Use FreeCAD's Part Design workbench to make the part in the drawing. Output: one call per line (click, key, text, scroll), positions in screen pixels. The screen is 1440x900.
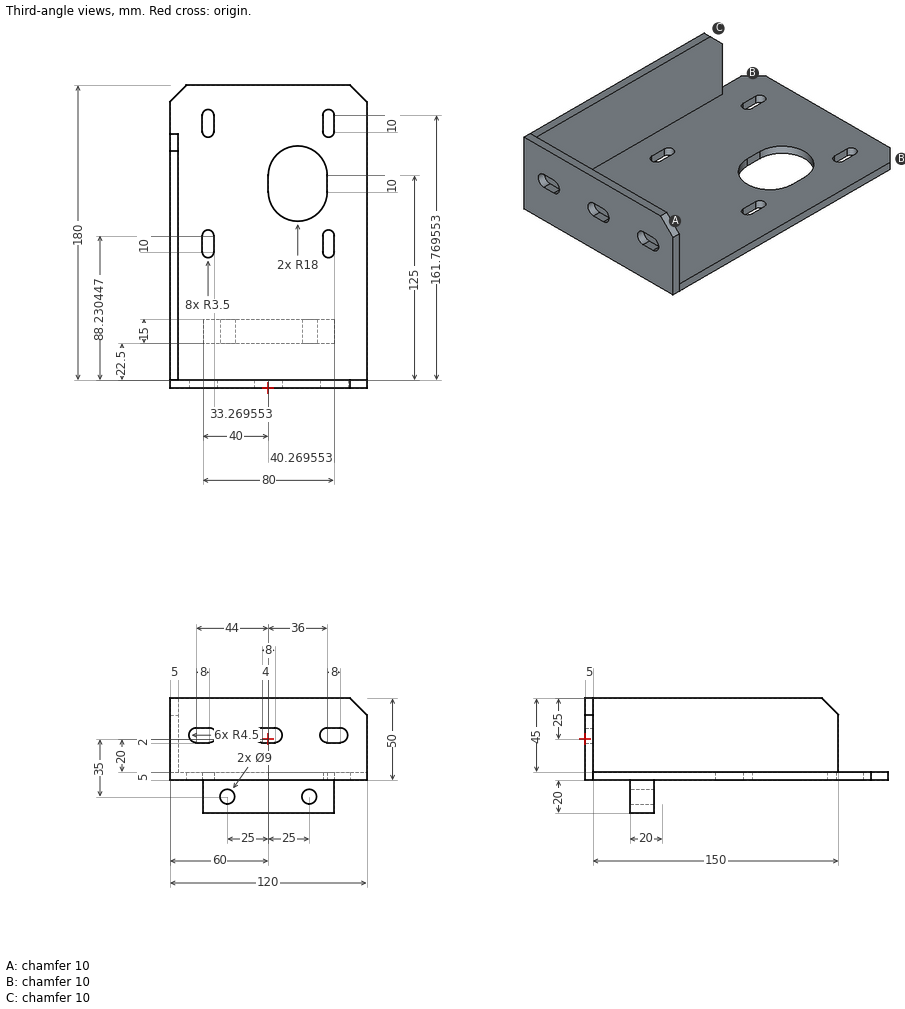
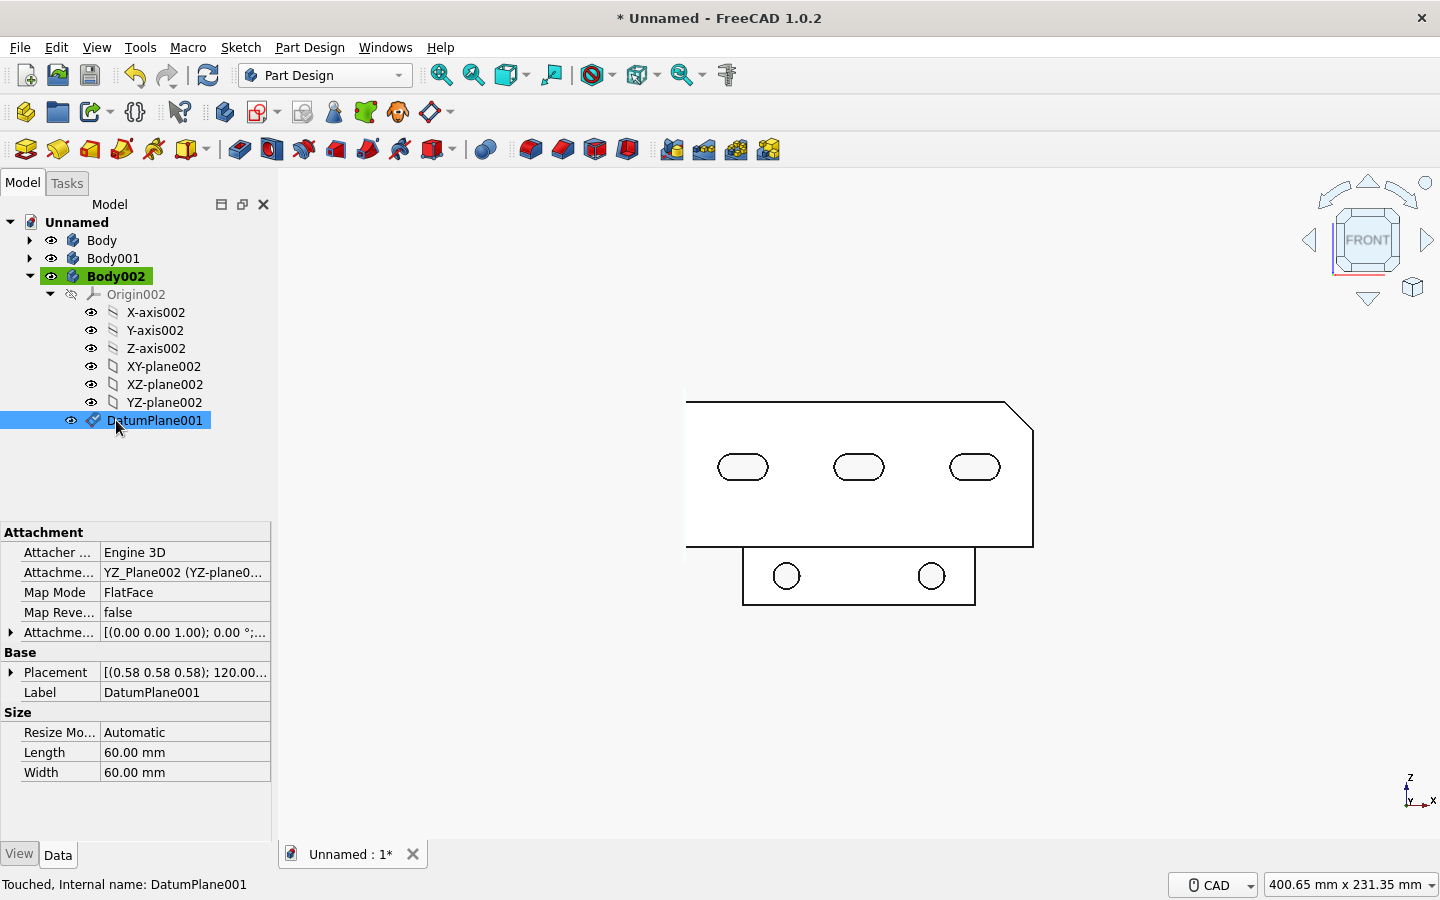
click(258, 112)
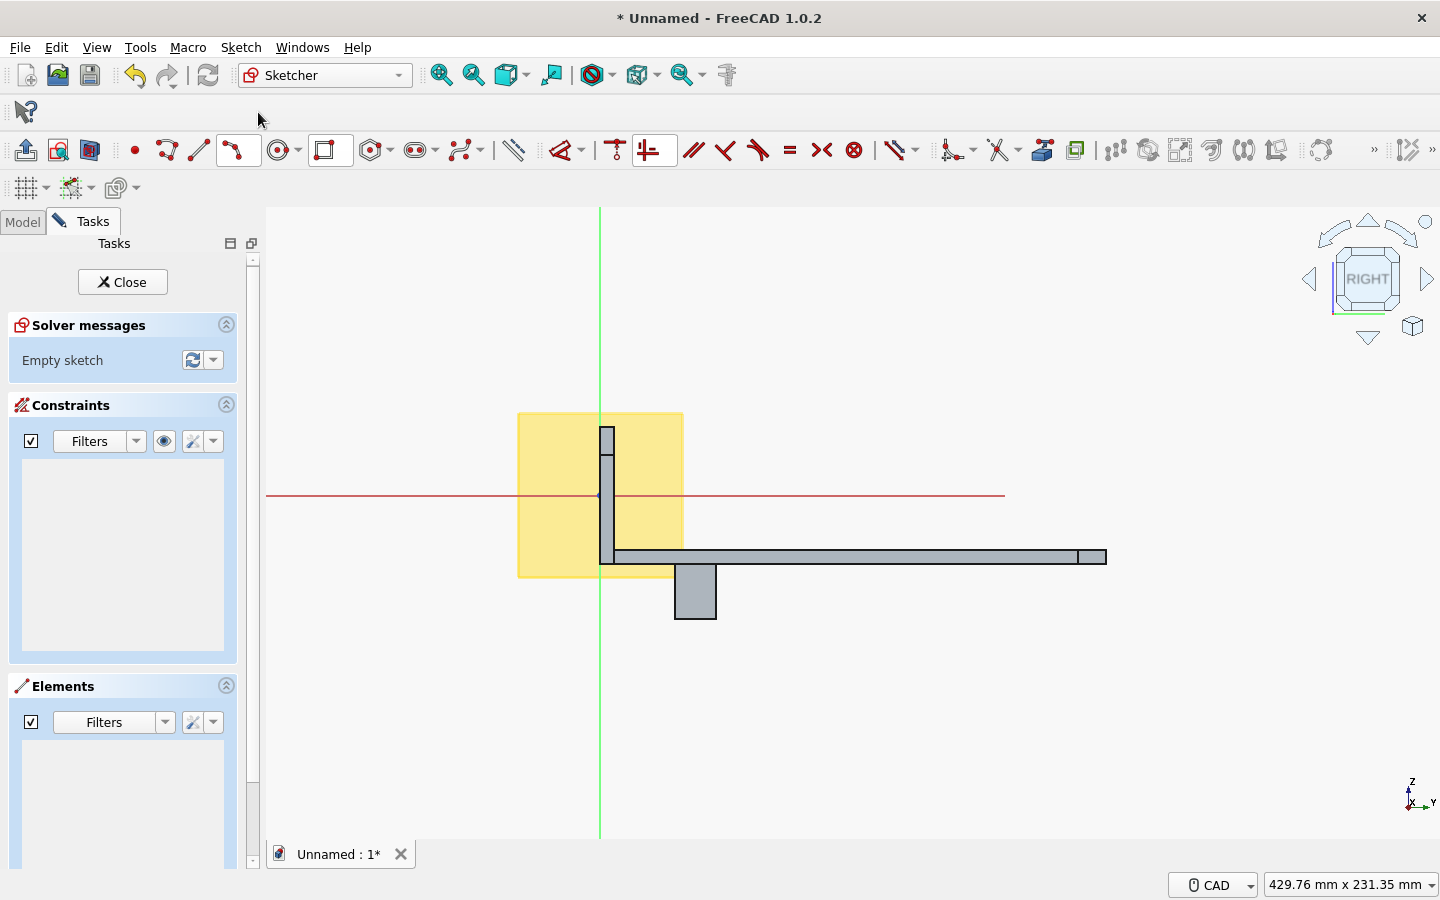
scroll(868, 419, up, 2)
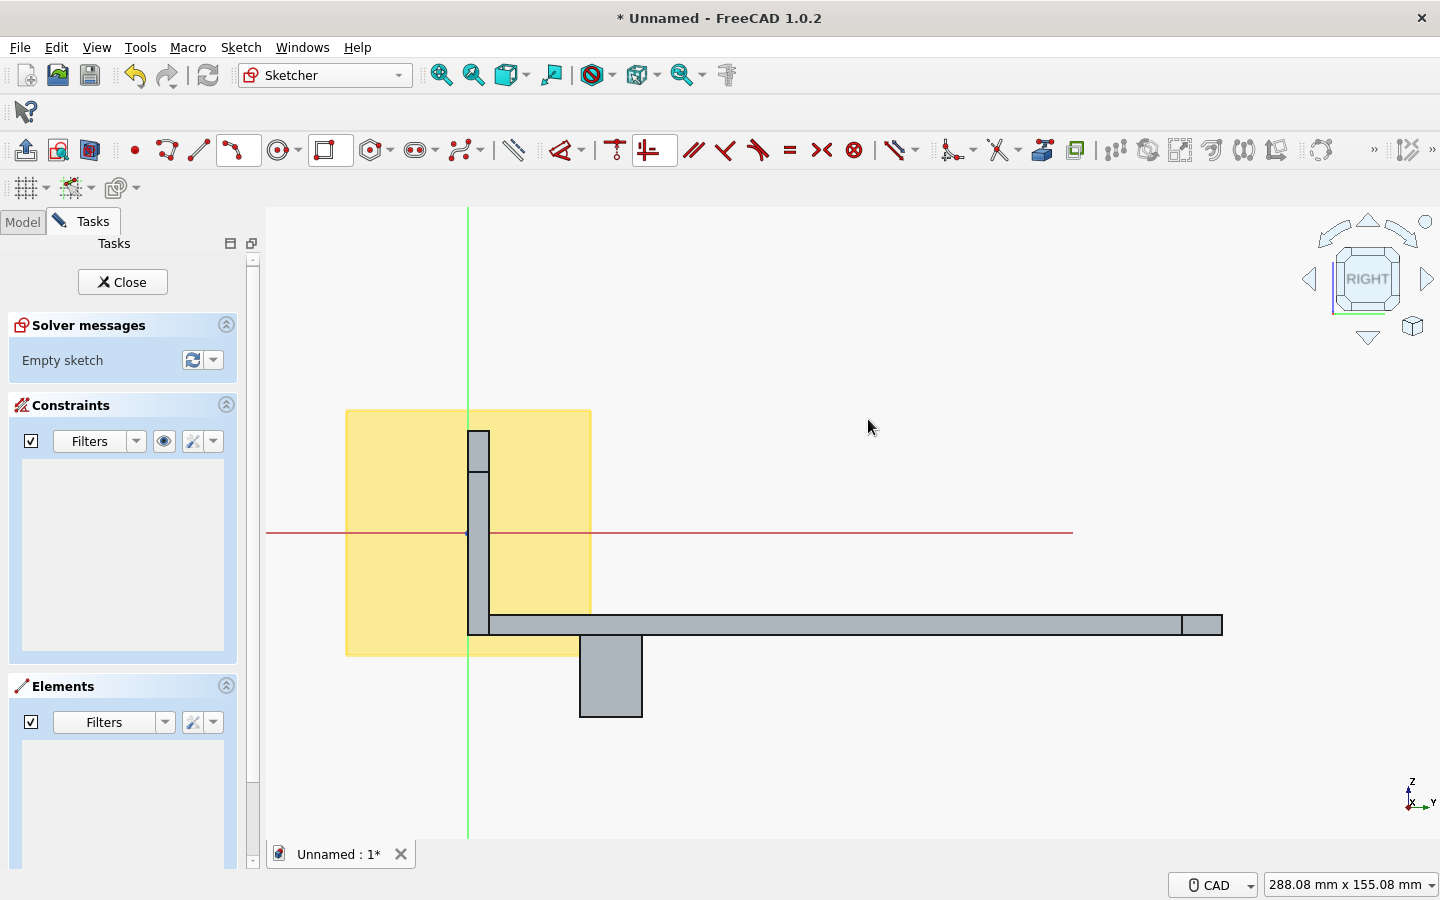
key(g)
key(r)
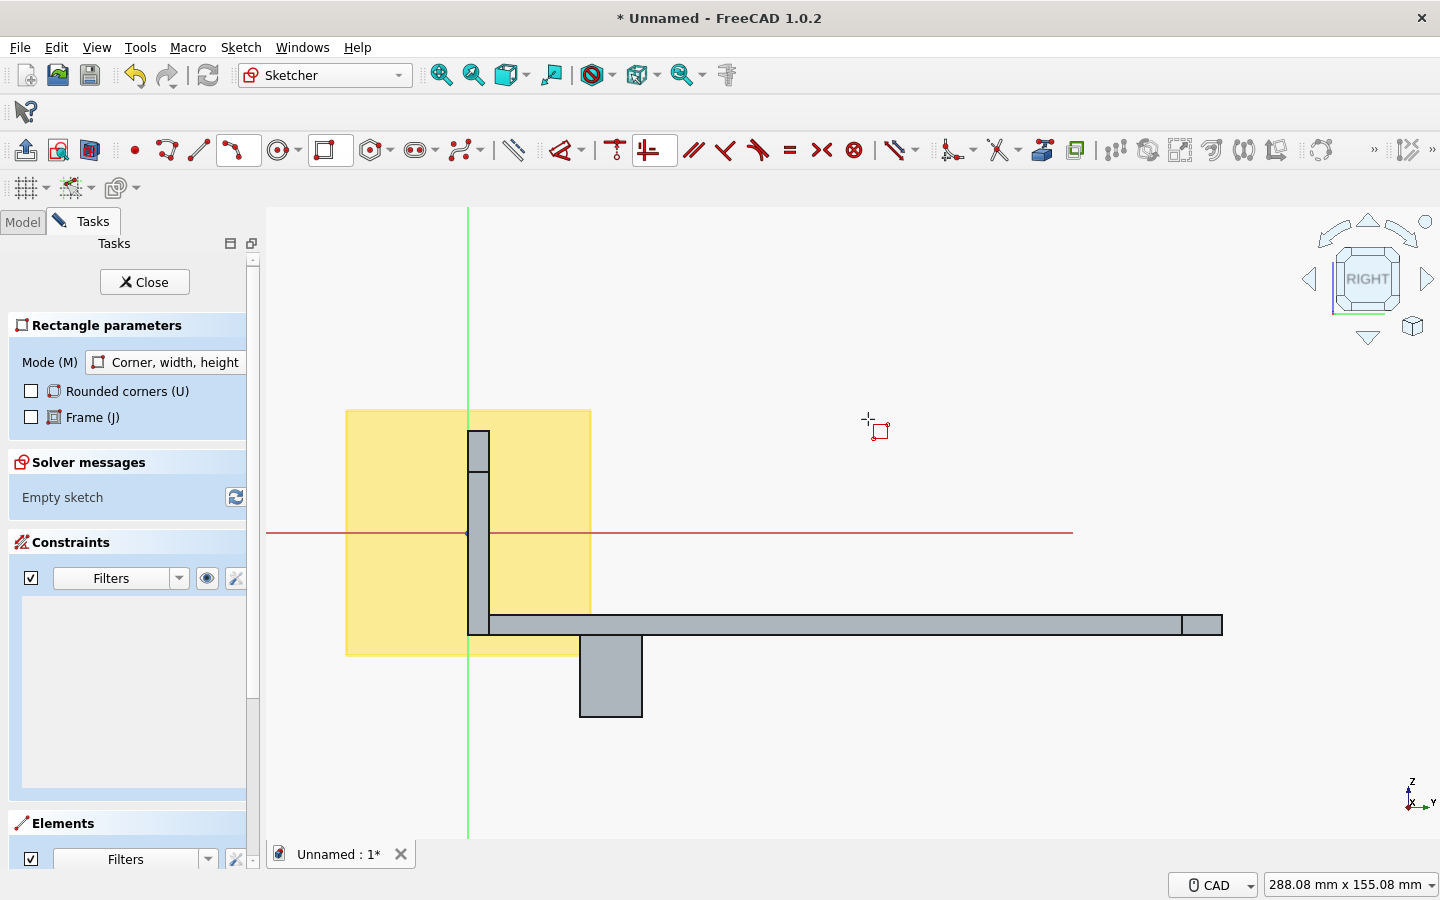
click(489, 431)
click(1100, 615)
key(Escape)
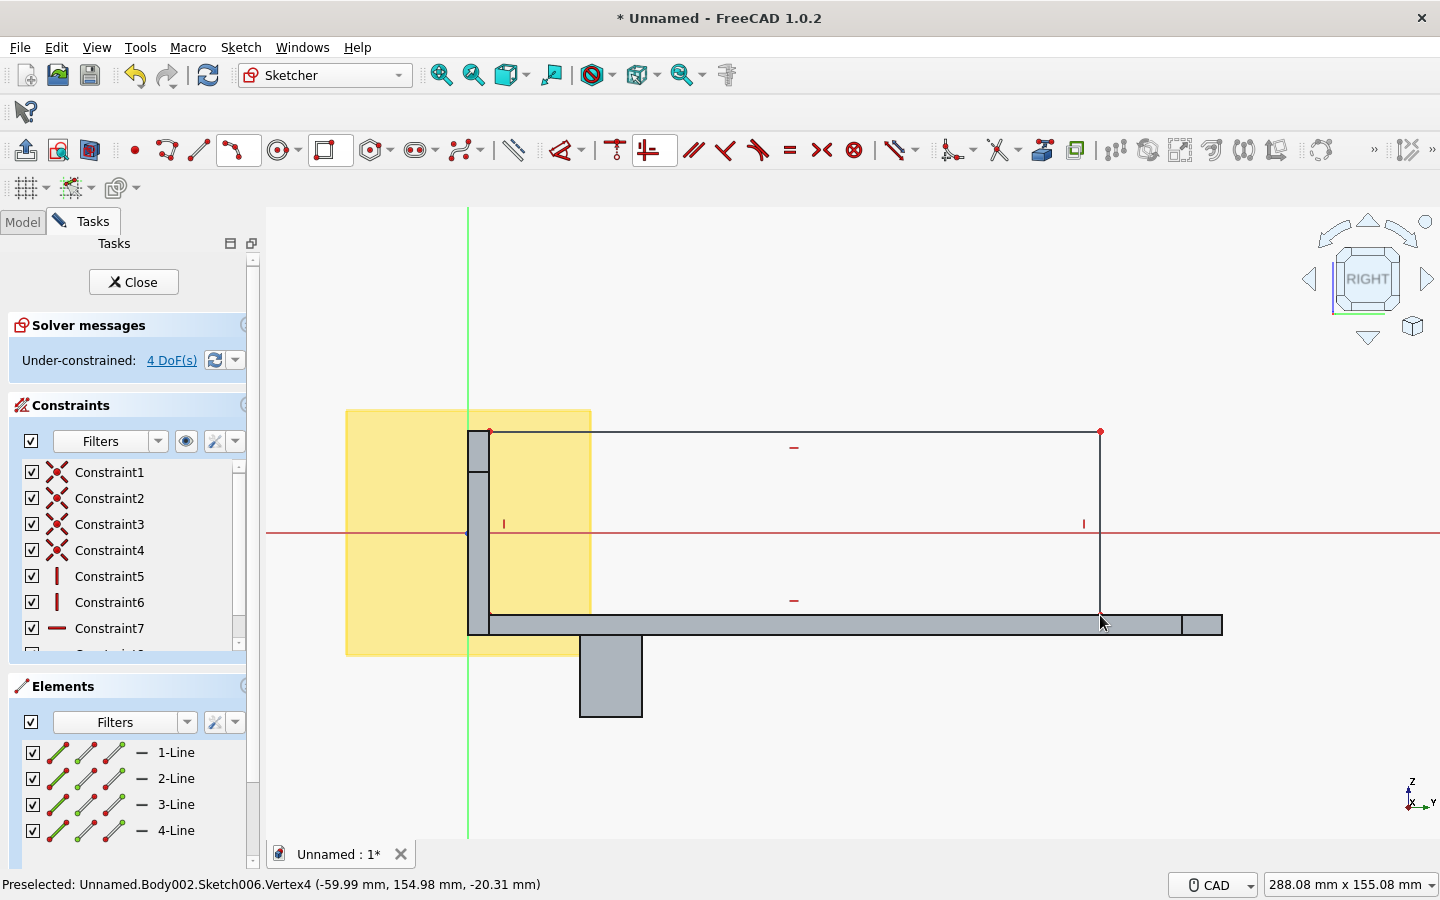
key(d)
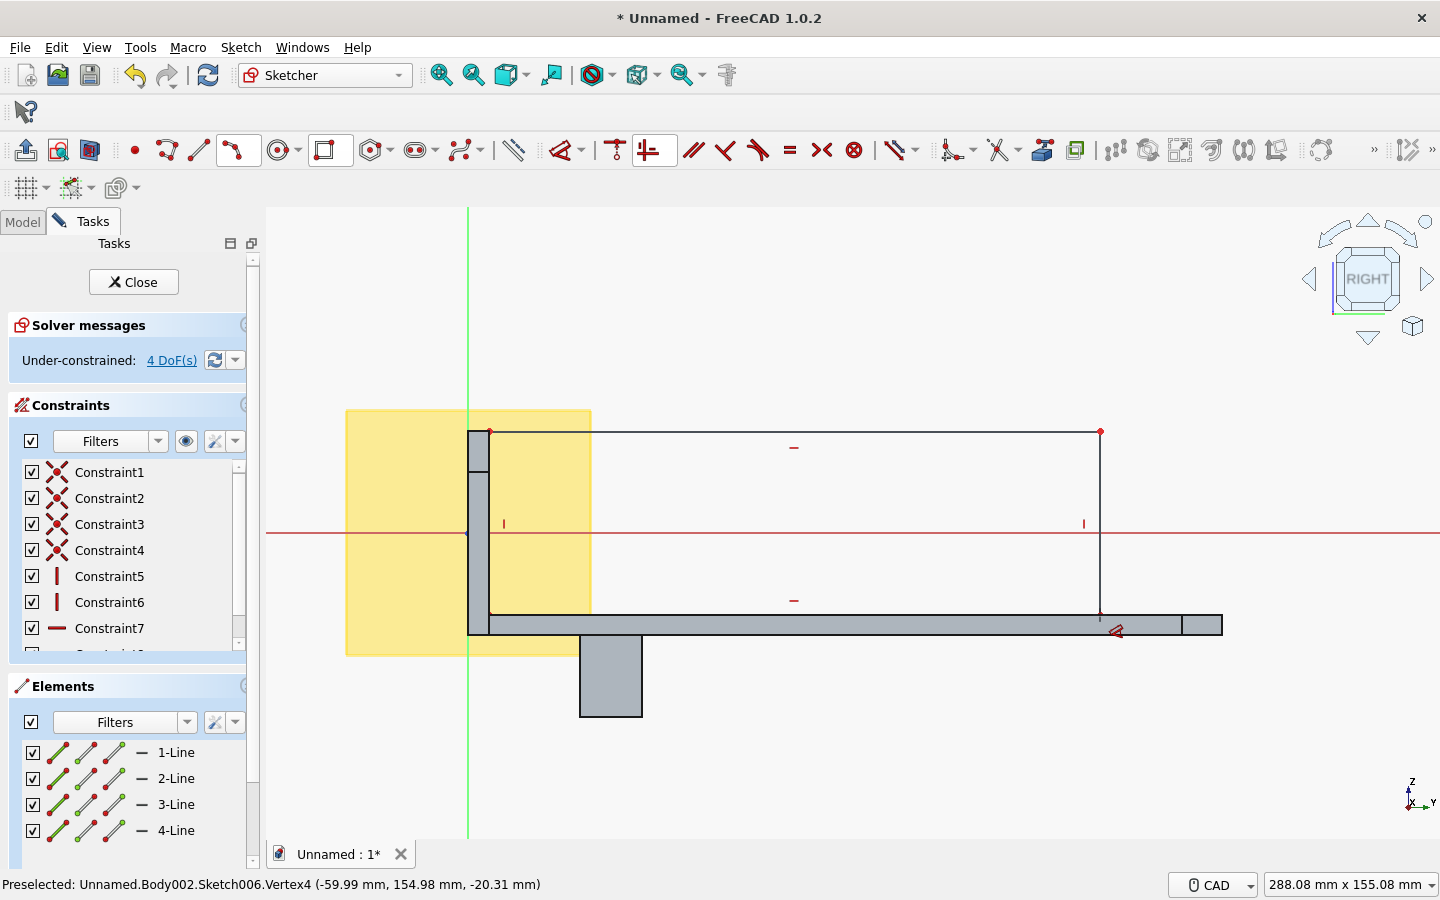
click(489, 487)
click(455, 482)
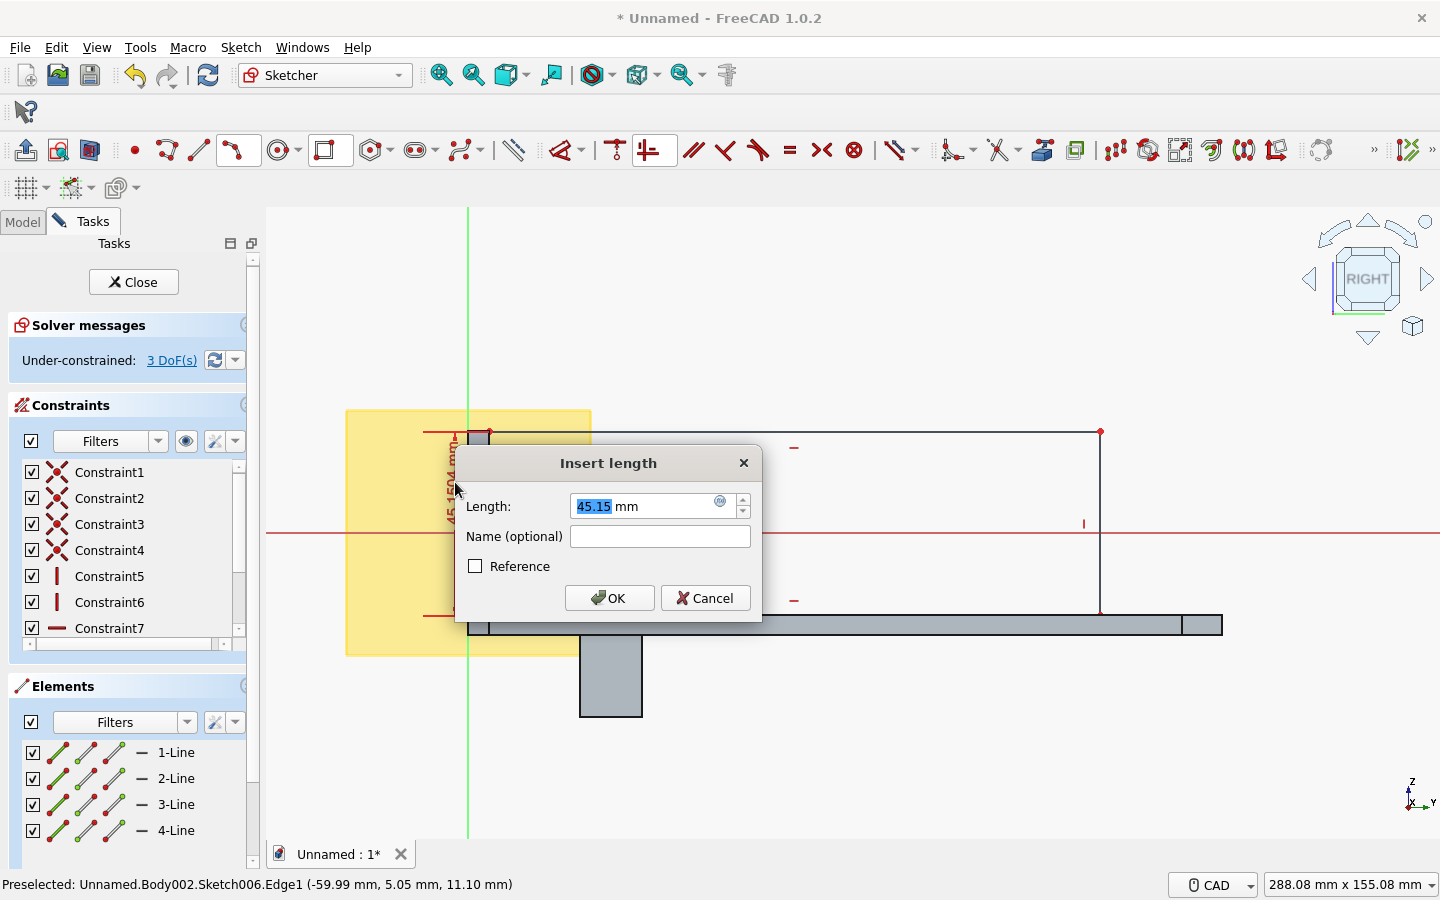
text(45)
key(Return)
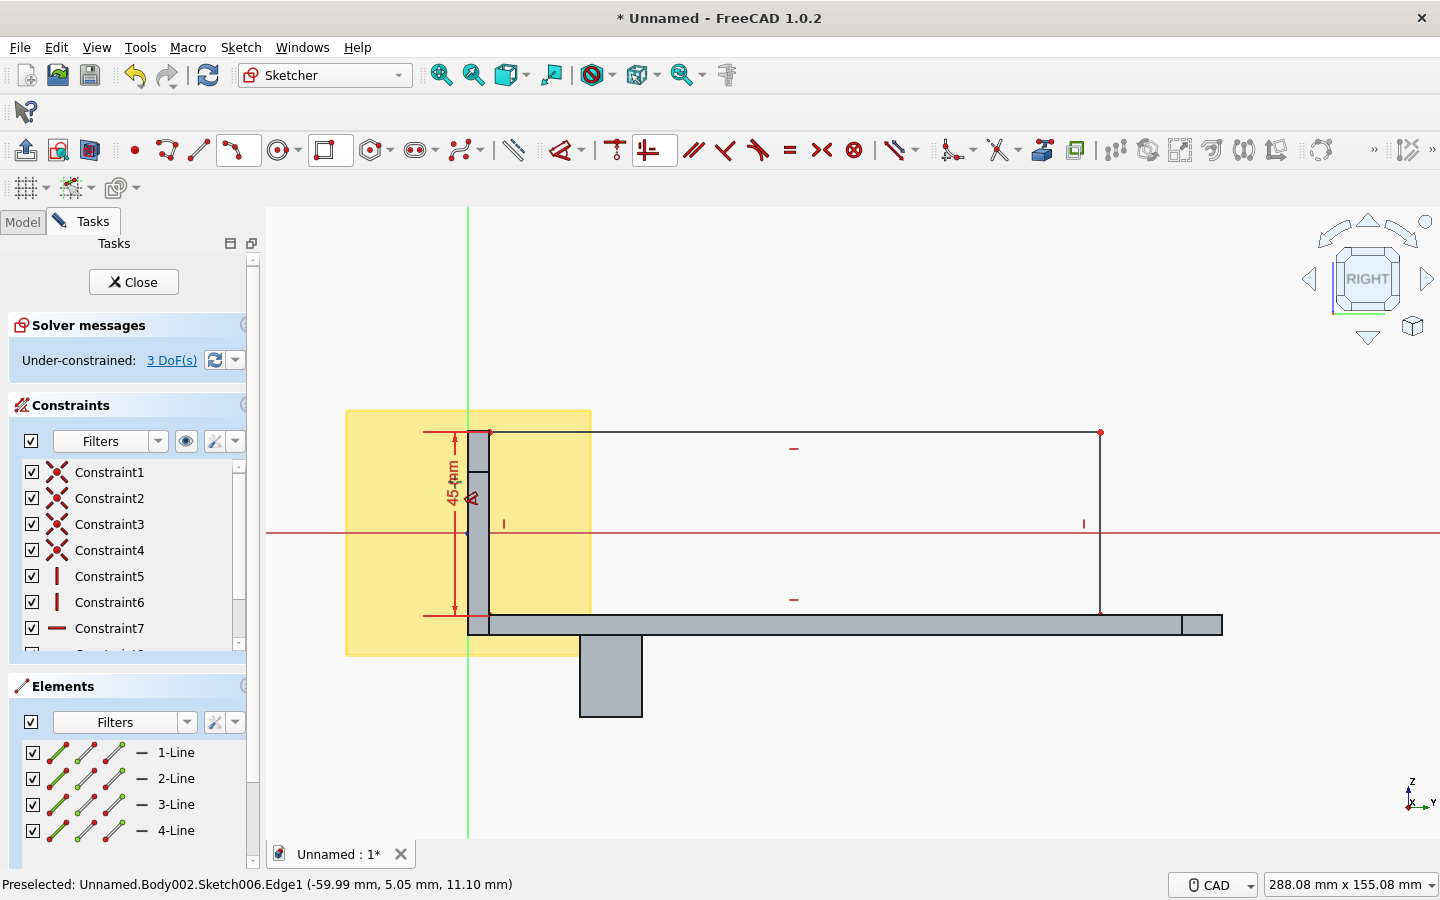
scroll(489, 432, up, 4)